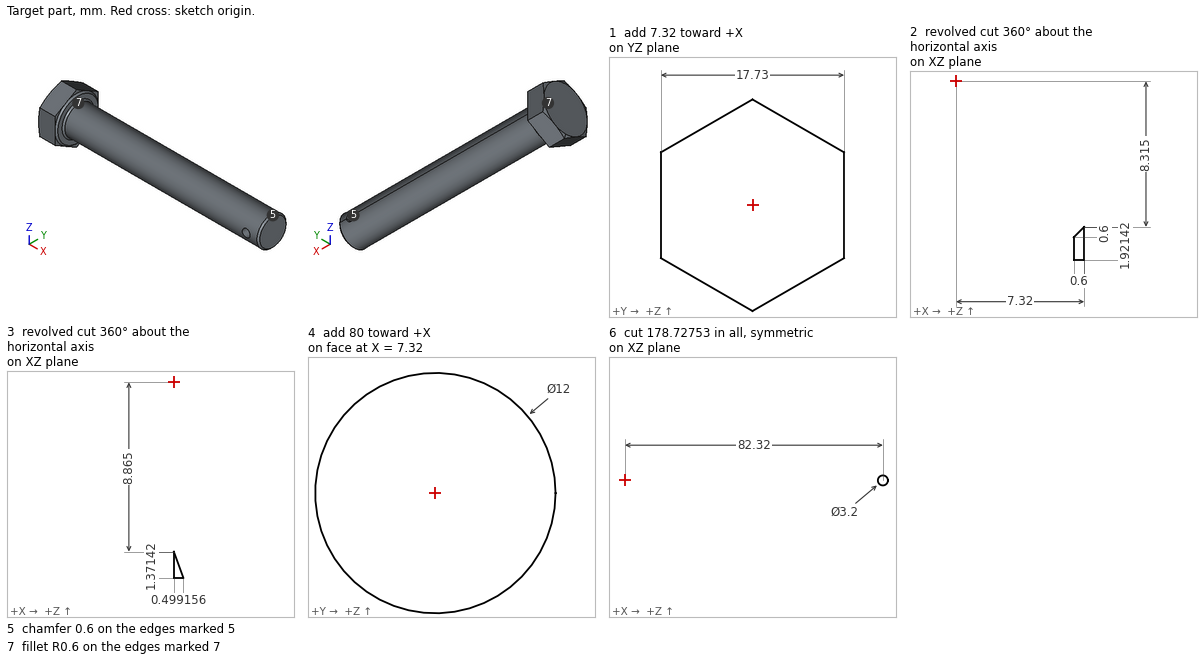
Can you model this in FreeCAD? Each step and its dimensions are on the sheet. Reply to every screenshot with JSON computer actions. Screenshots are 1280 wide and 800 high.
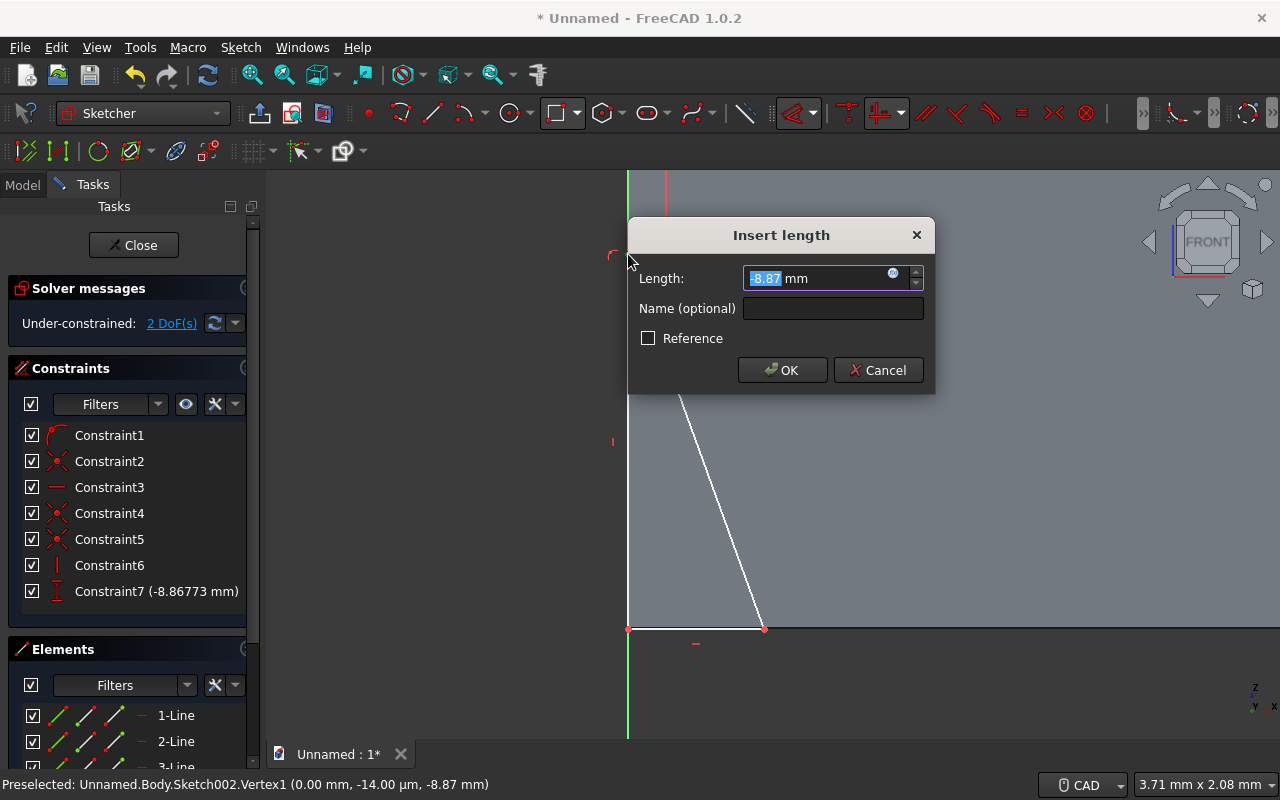
{"action": "type", "text": "-8.865"}
{"action": "key", "text": "Return"}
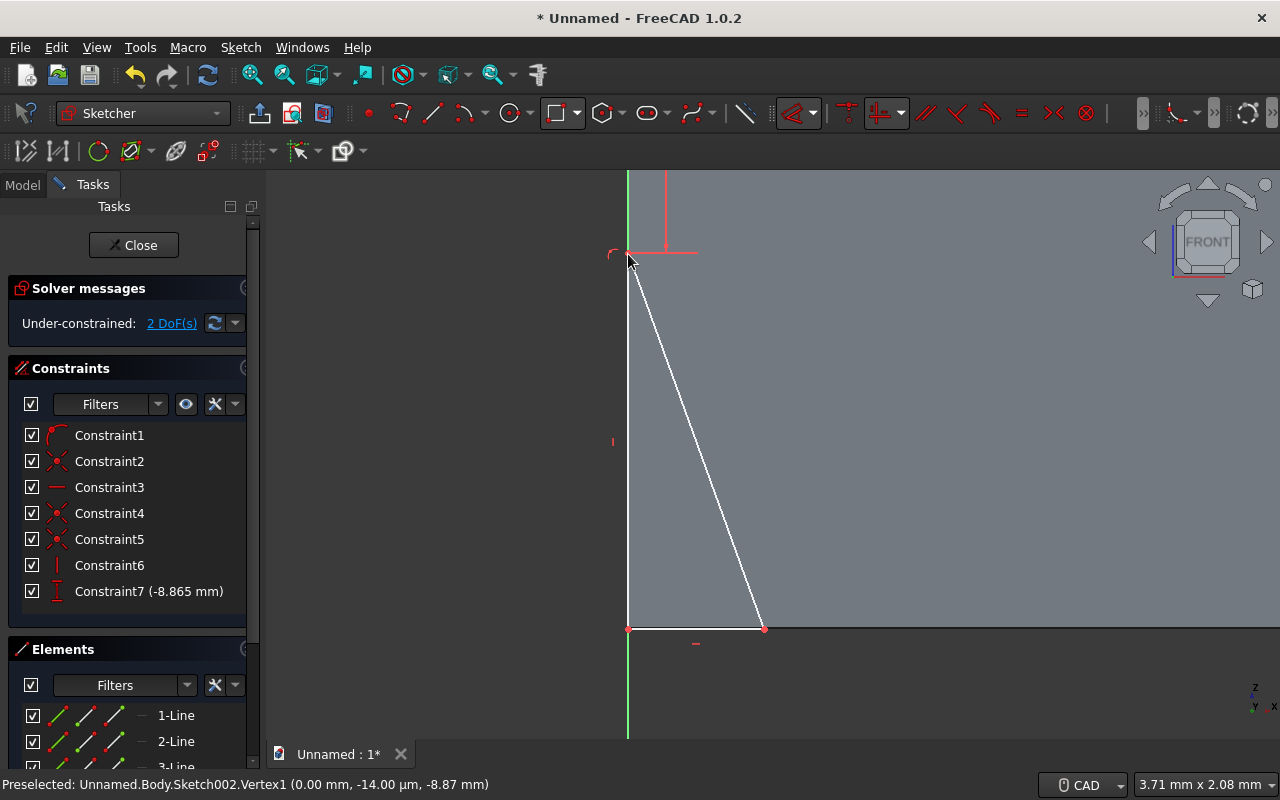
{"action": "left_click", "coordinate": [628, 516]}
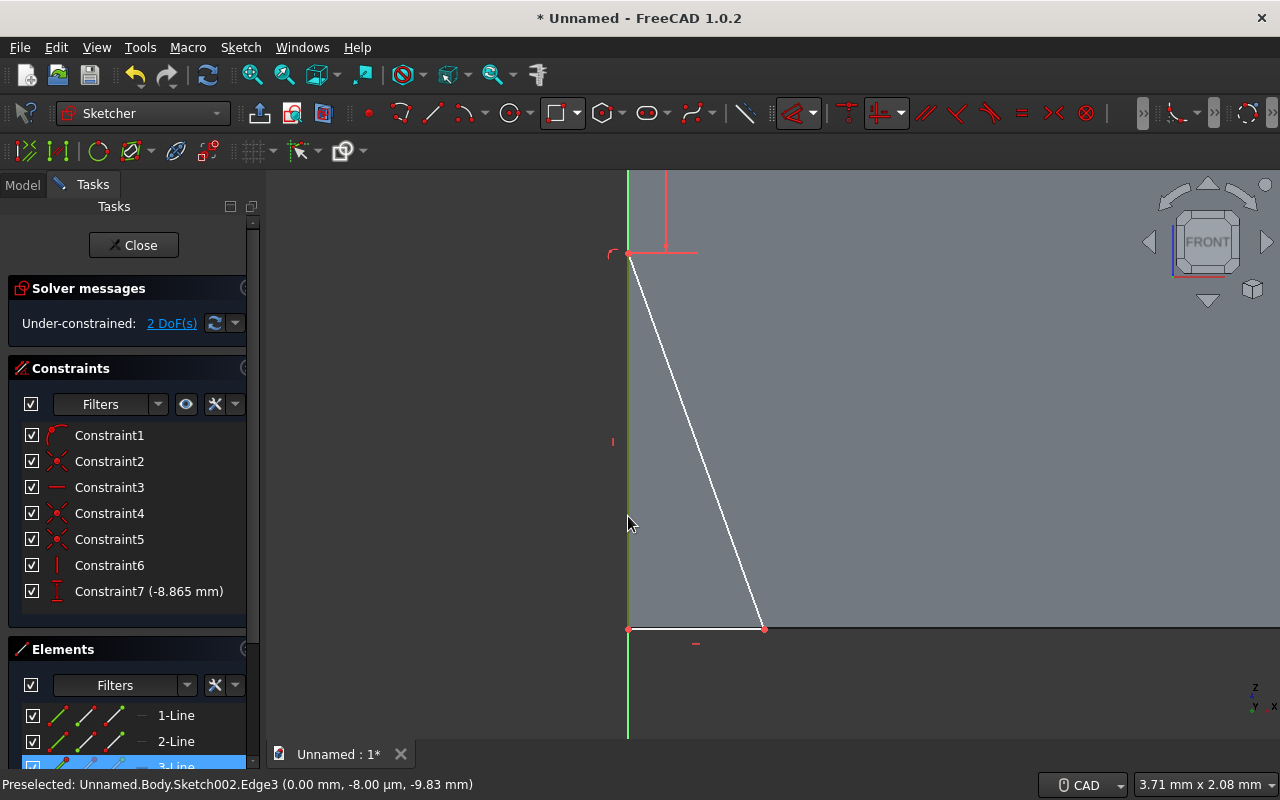
{"action": "key", "text": "i"}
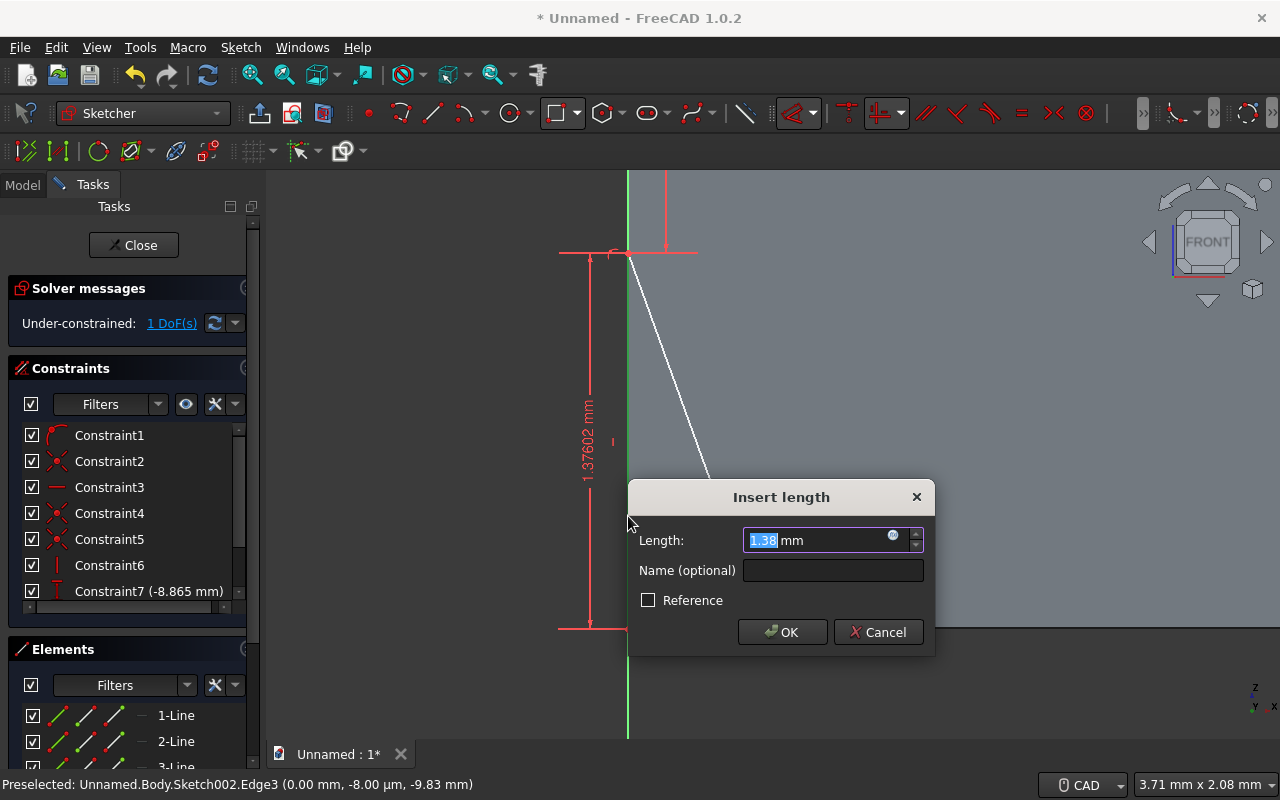
{"action": "type", "text": "1.37142"}
{"action": "key", "text": "Return"}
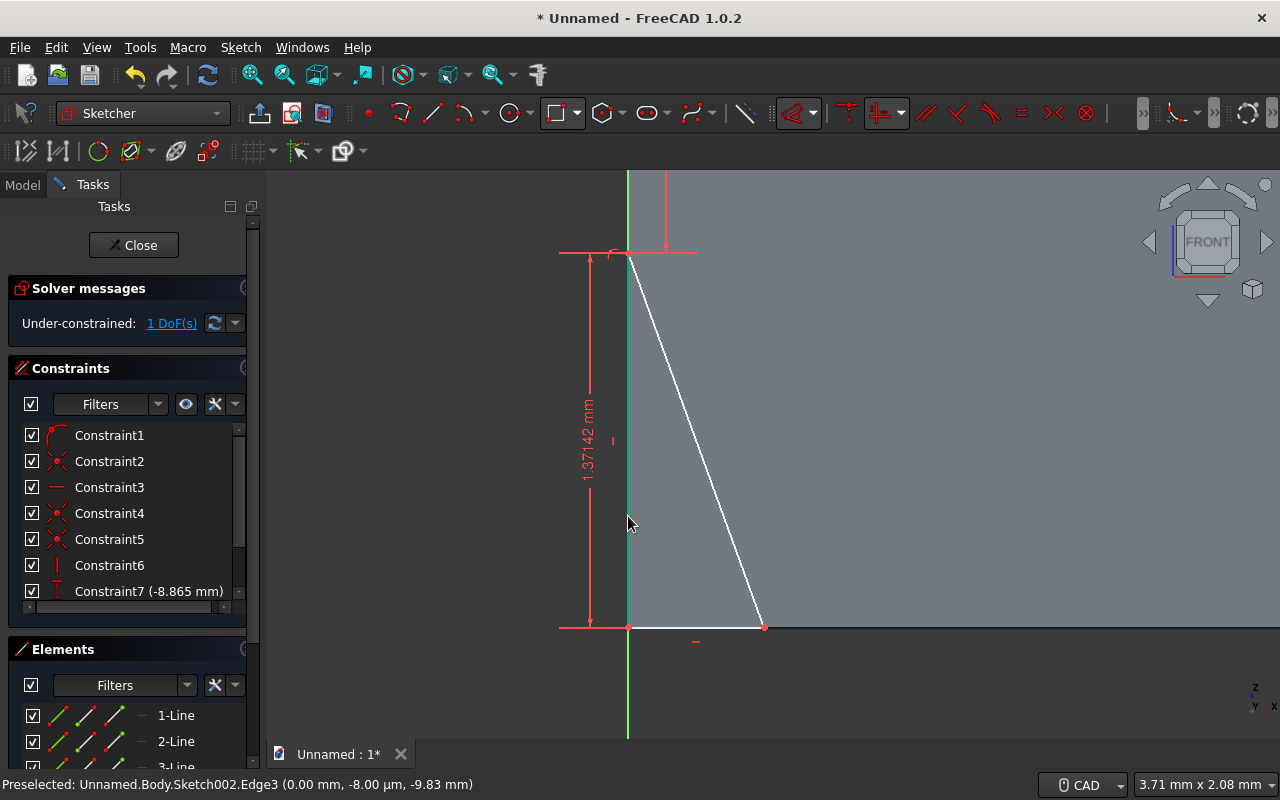
{"action": "left_click", "coordinate": [723, 628]}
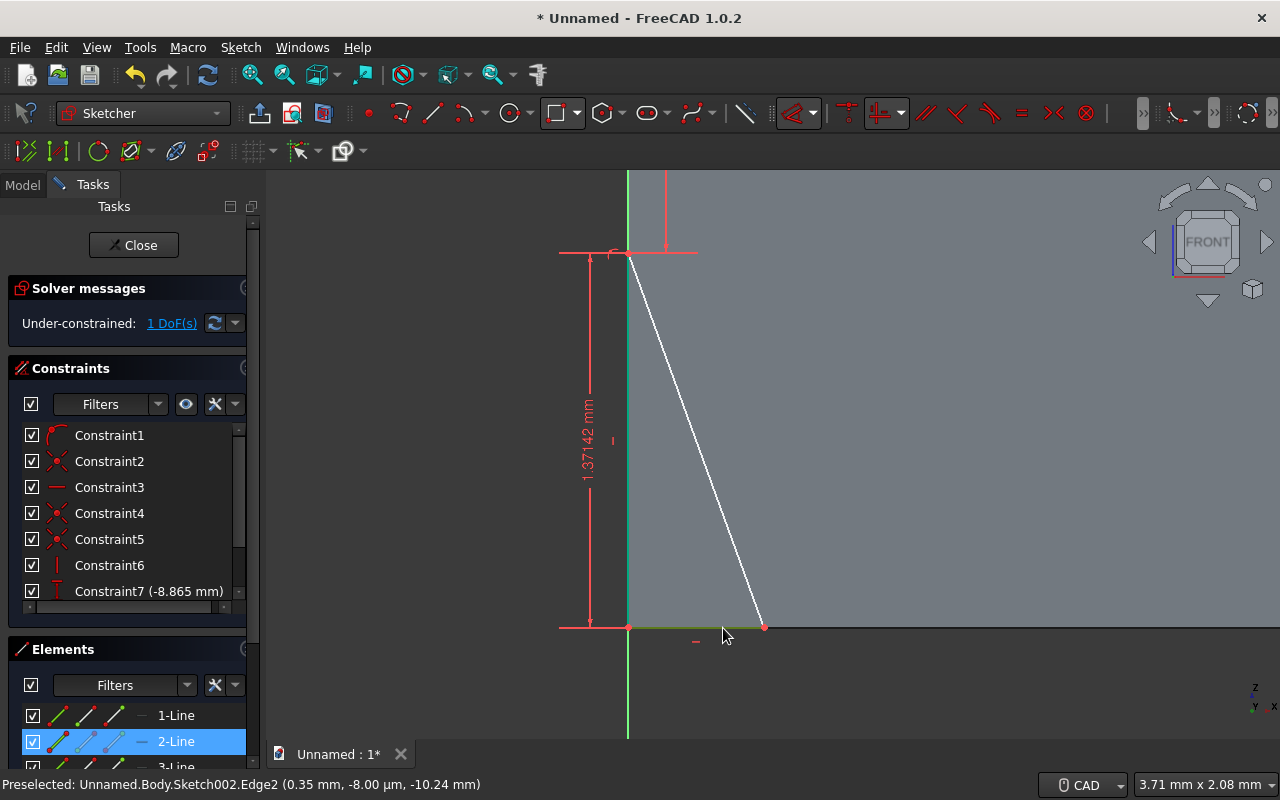
{"action": "left_click", "coordinate": [816, 114]}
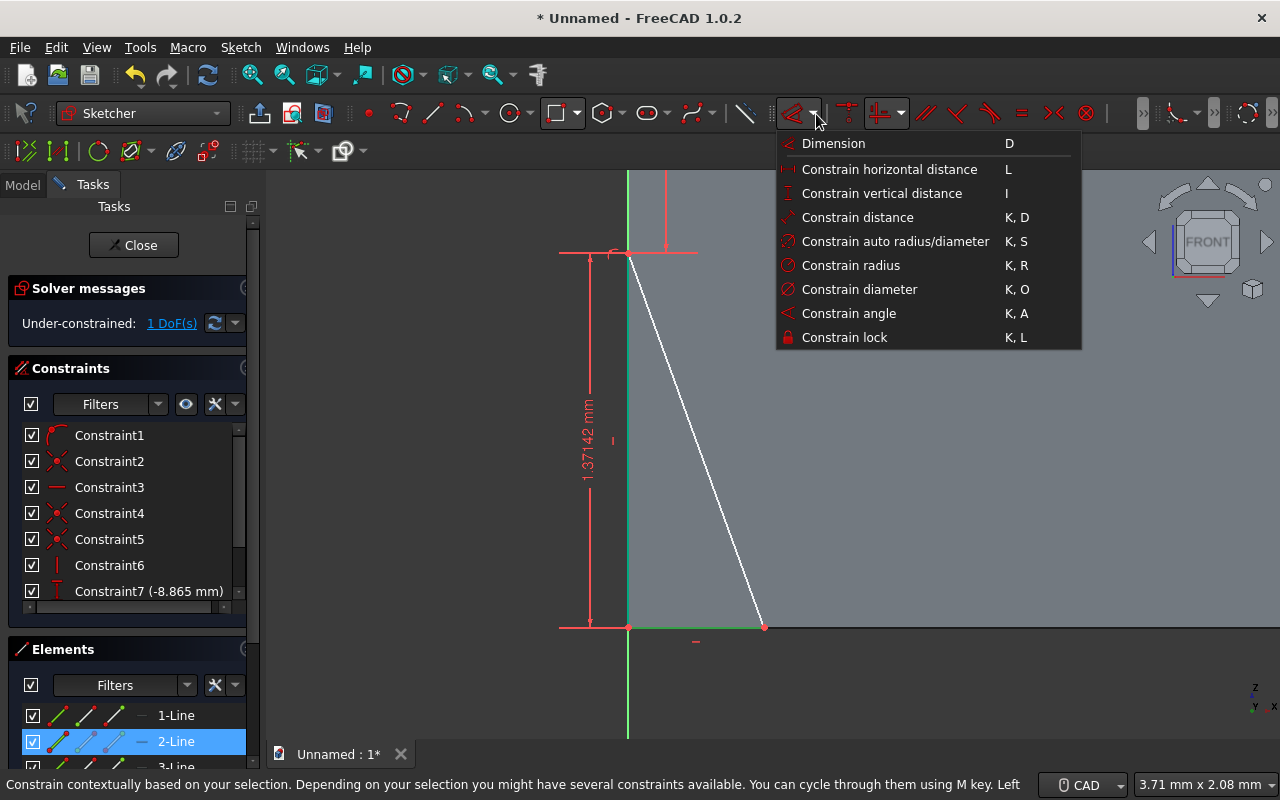
{"action": "left_click", "coordinate": [929, 169]}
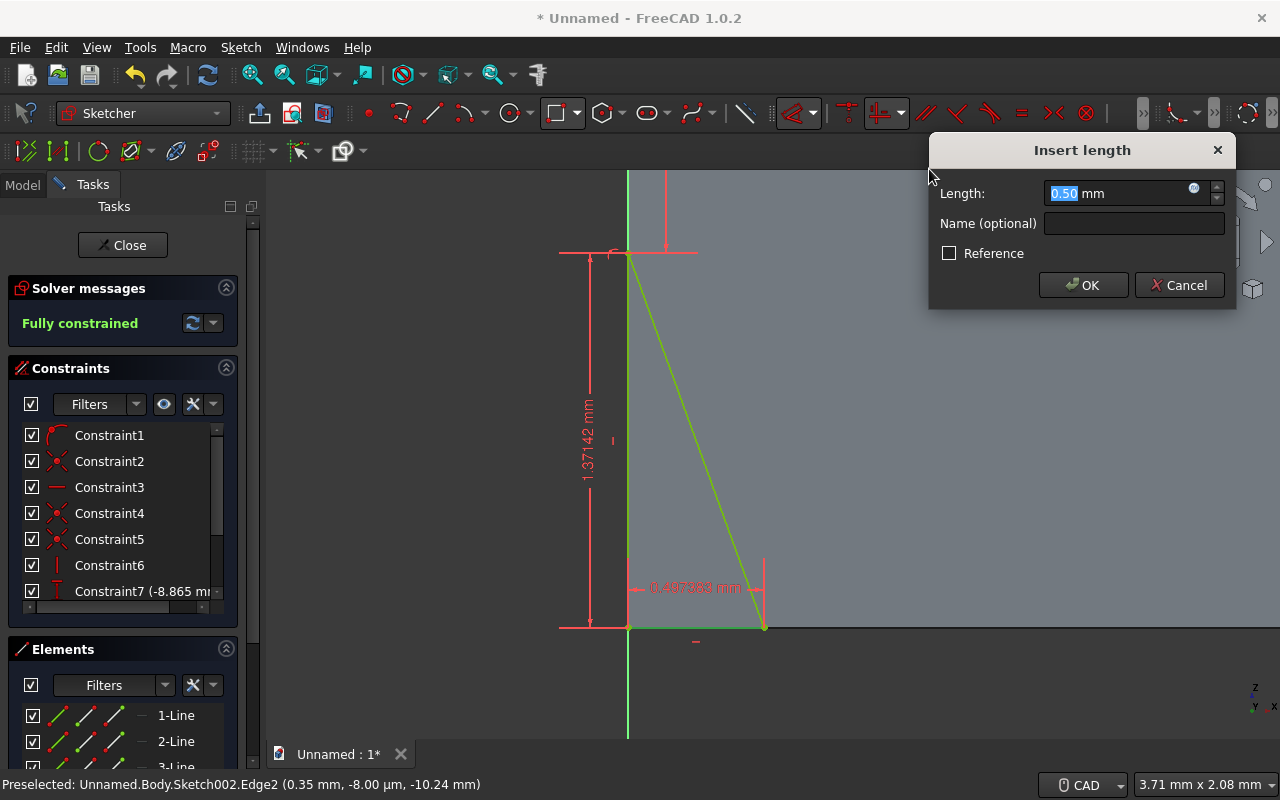
{"action": "type", "text": "0.499156"}
{"action": "key", "text": "Return"}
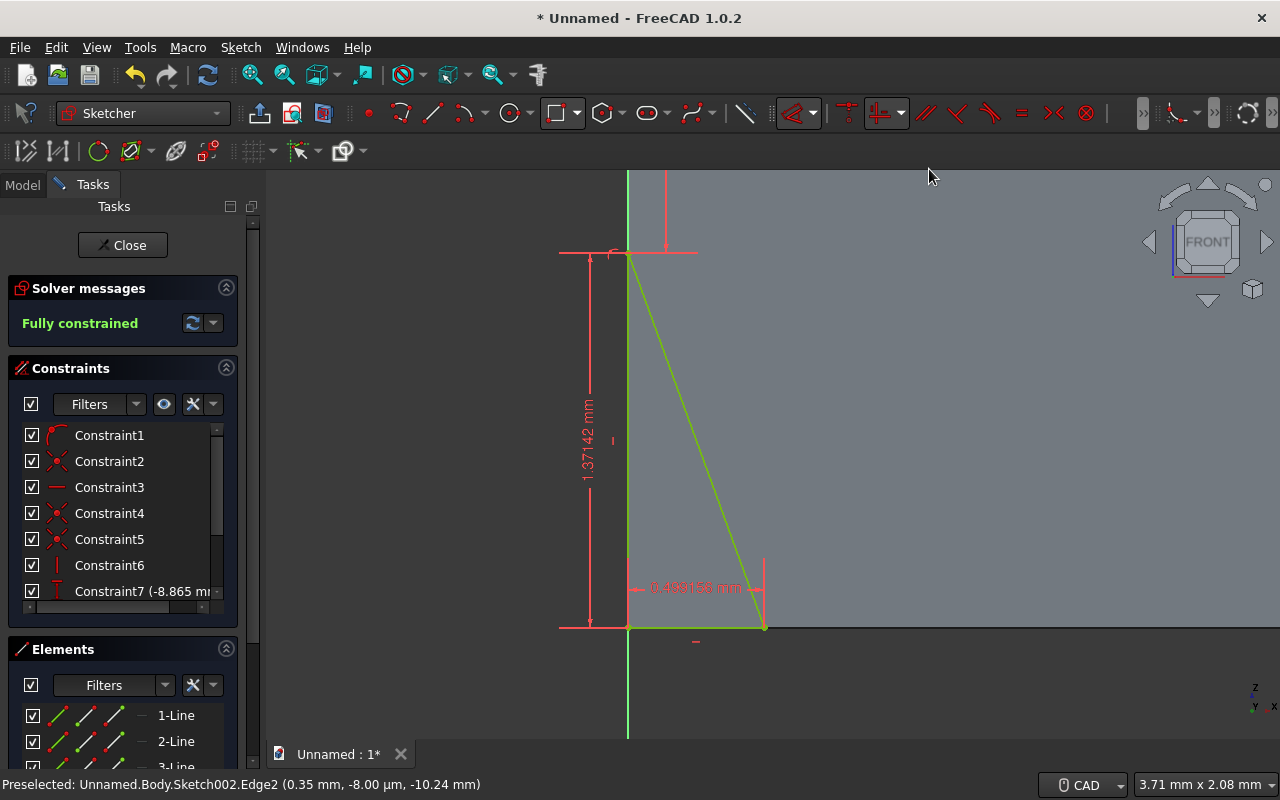
{"action": "left_click", "coordinate": [123, 245]}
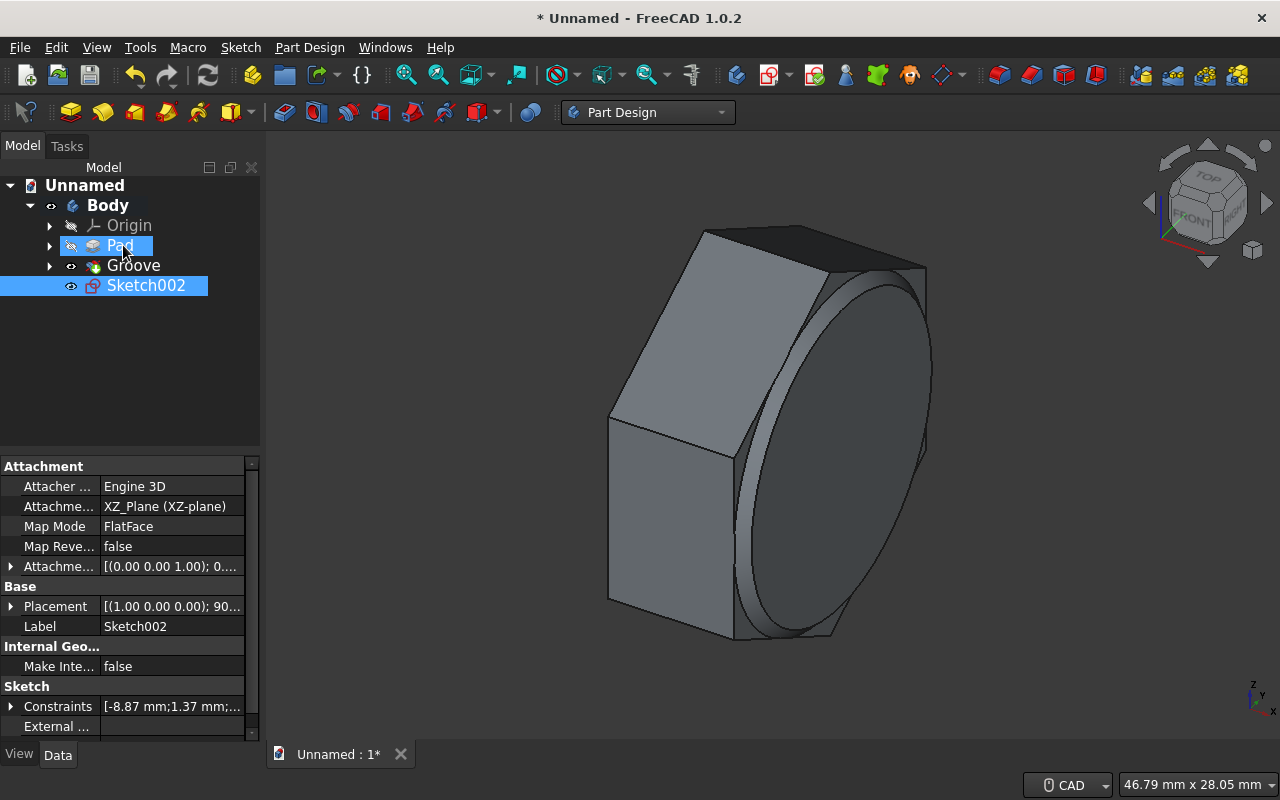
{"action": "left_click", "coordinate": [350, 112]}